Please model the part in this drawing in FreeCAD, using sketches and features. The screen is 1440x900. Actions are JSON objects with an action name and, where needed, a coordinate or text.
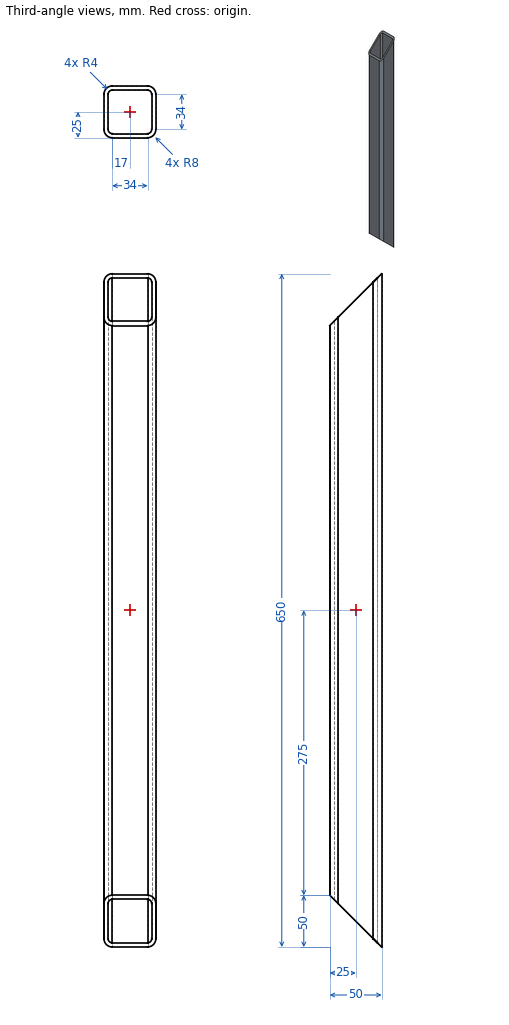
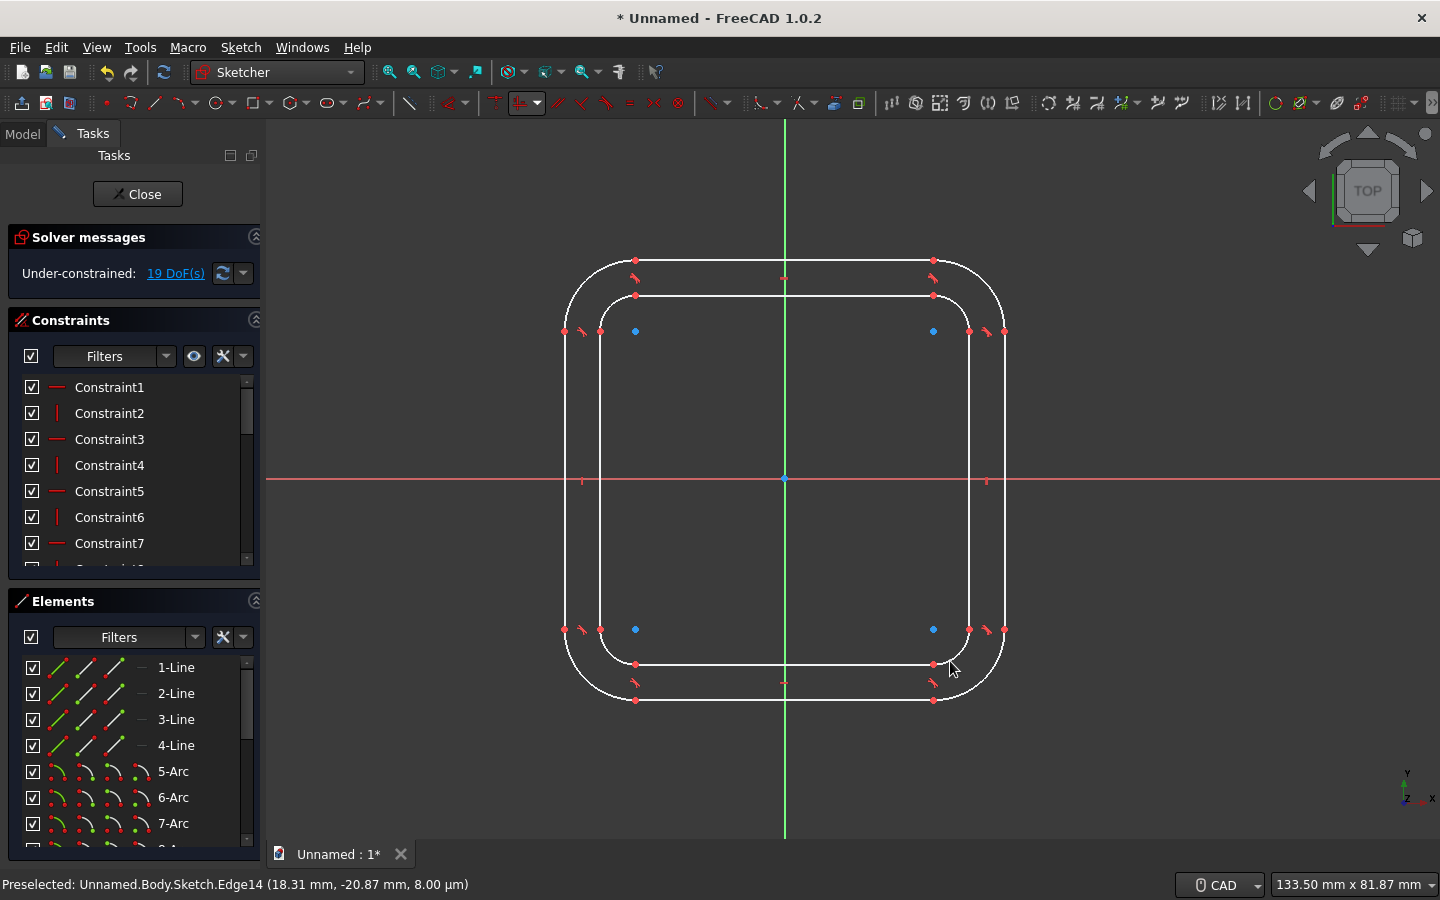
{"action": "left_click", "coordinate": [844, 665]}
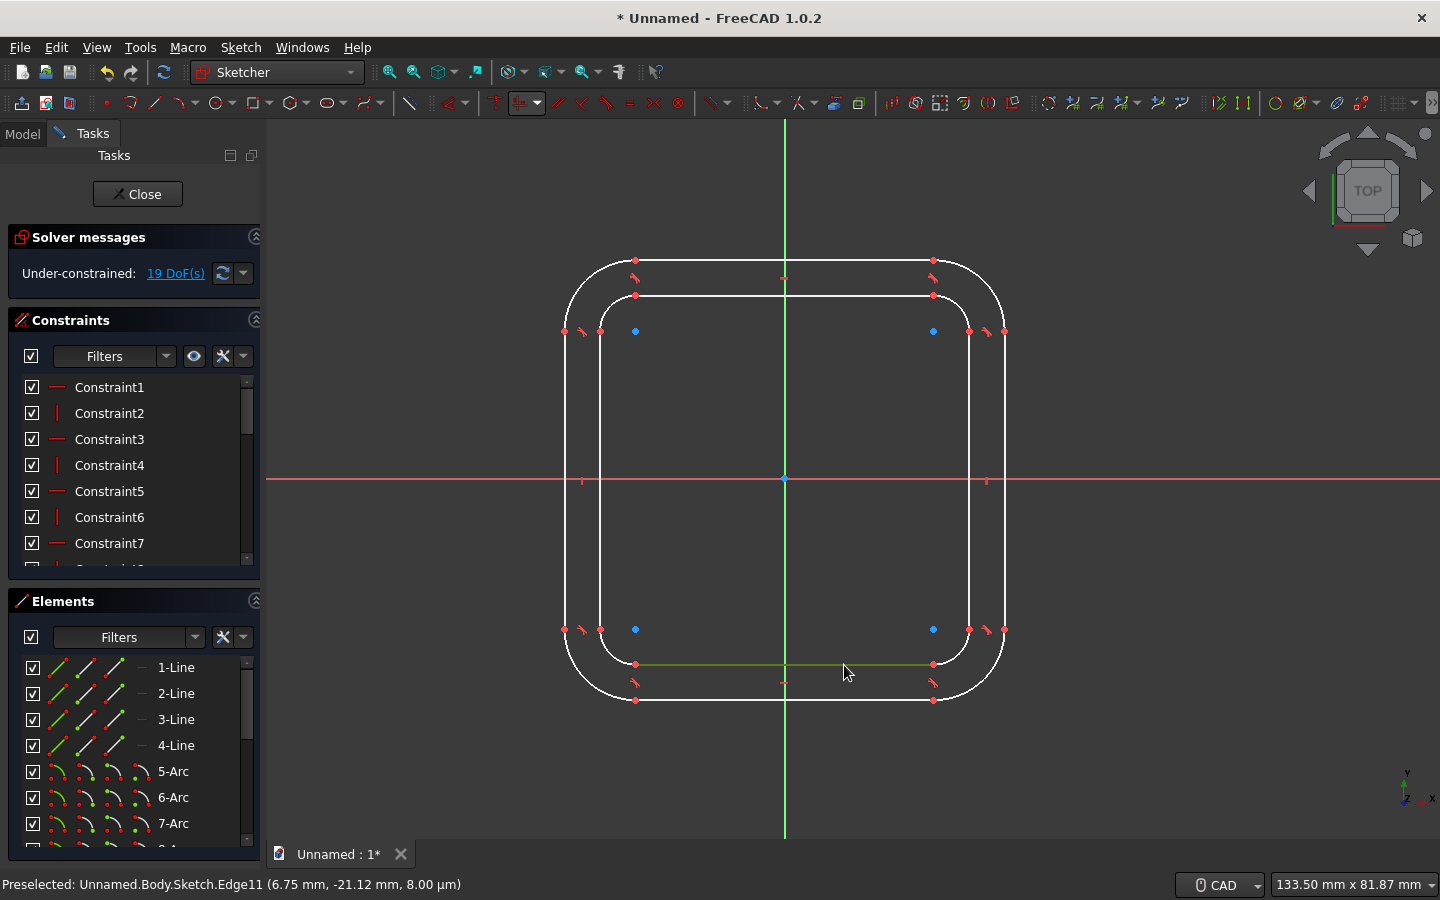
{"action": "left_click", "coordinate": [604, 645]}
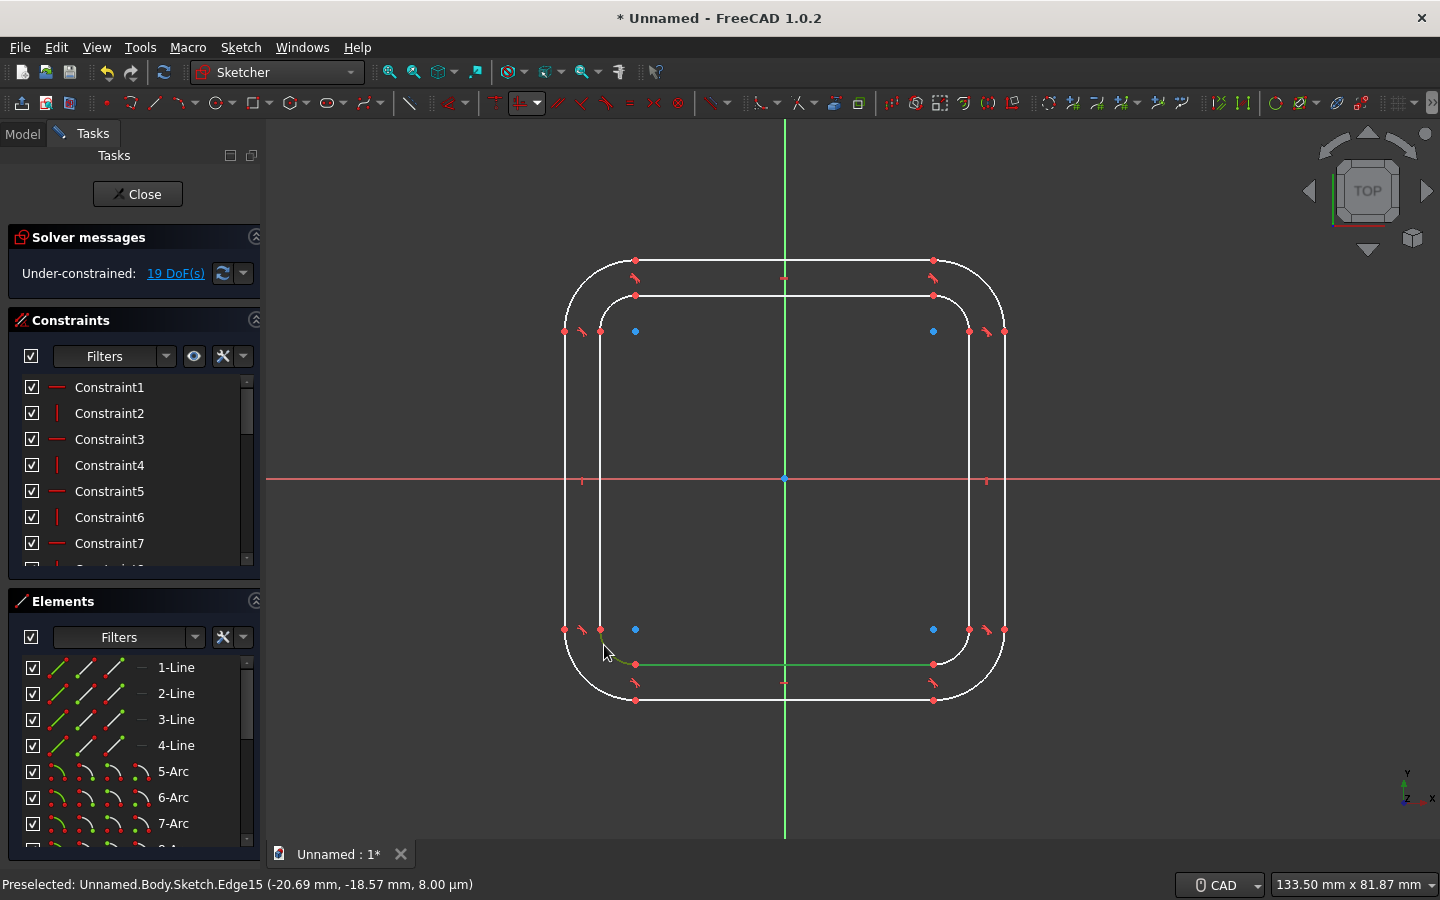
{"action": "left_click", "coordinate": [606, 104]}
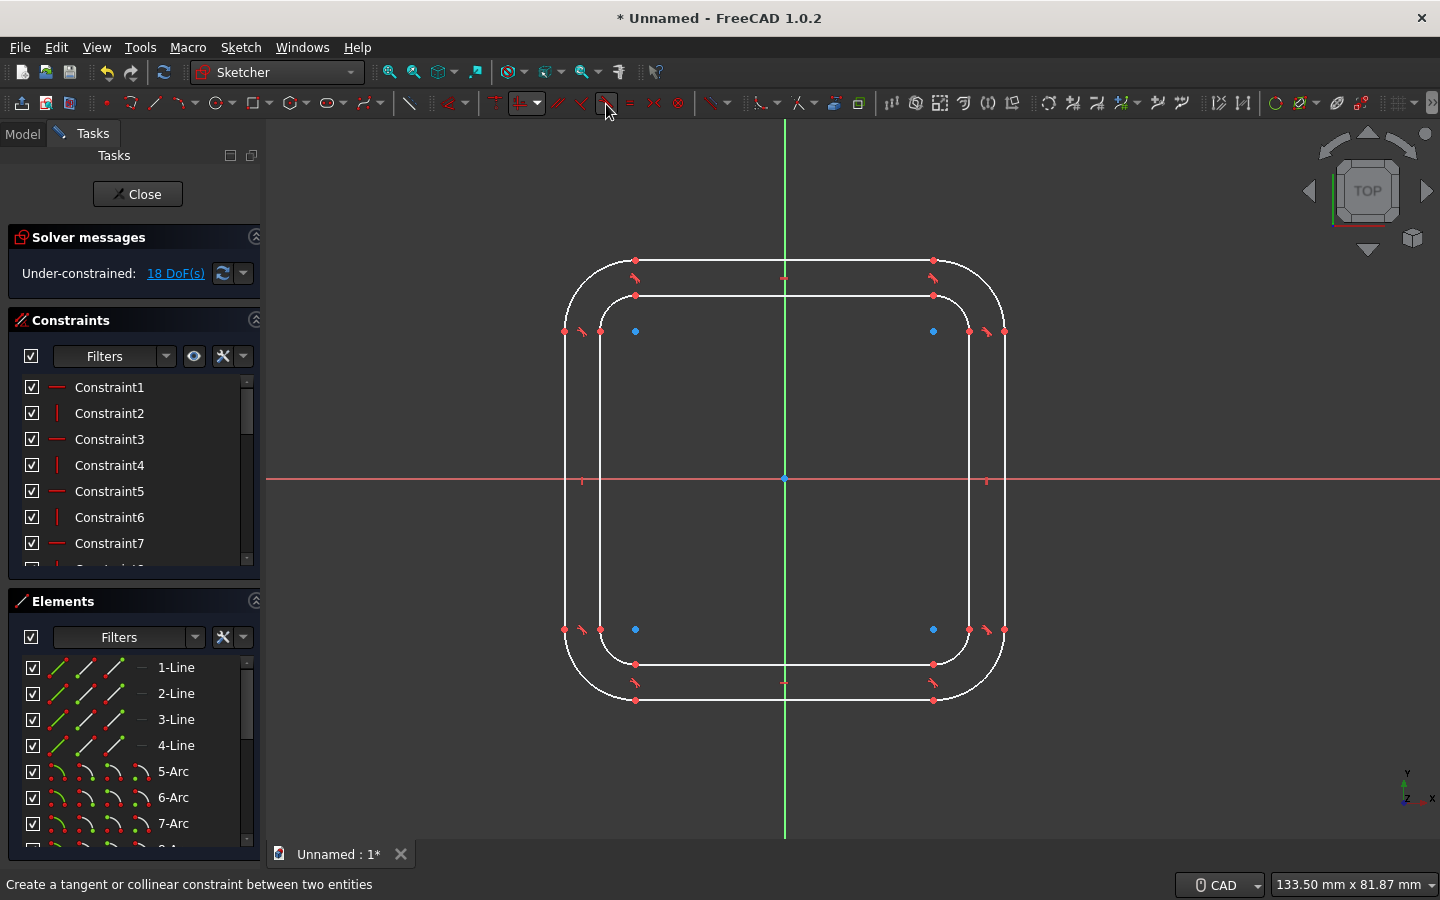
{"action": "left_click", "coordinate": [600, 540]}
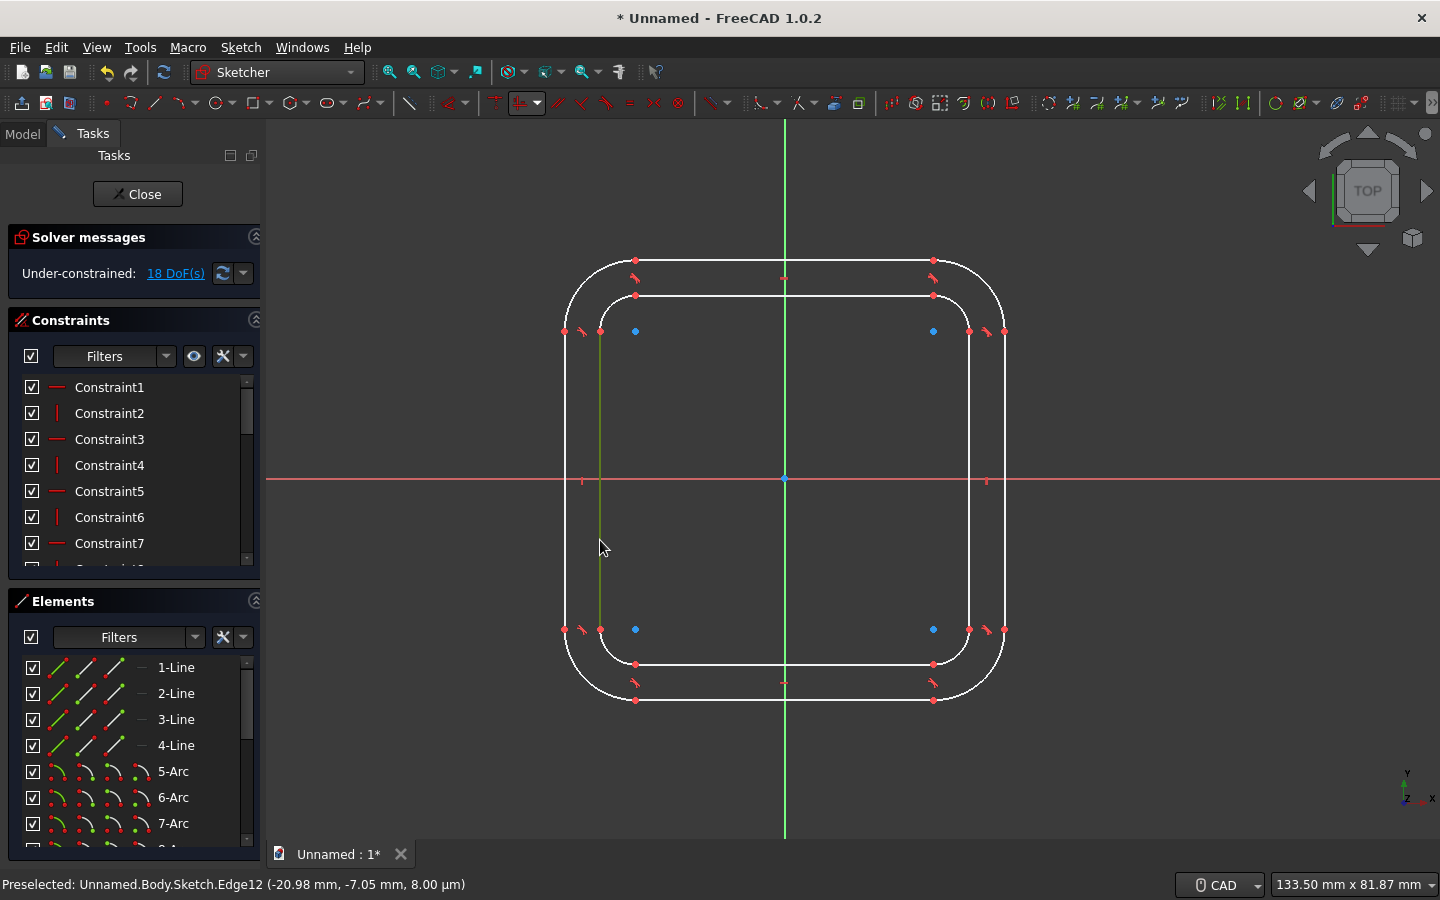
{"action": "left_click", "coordinate": [604, 645]}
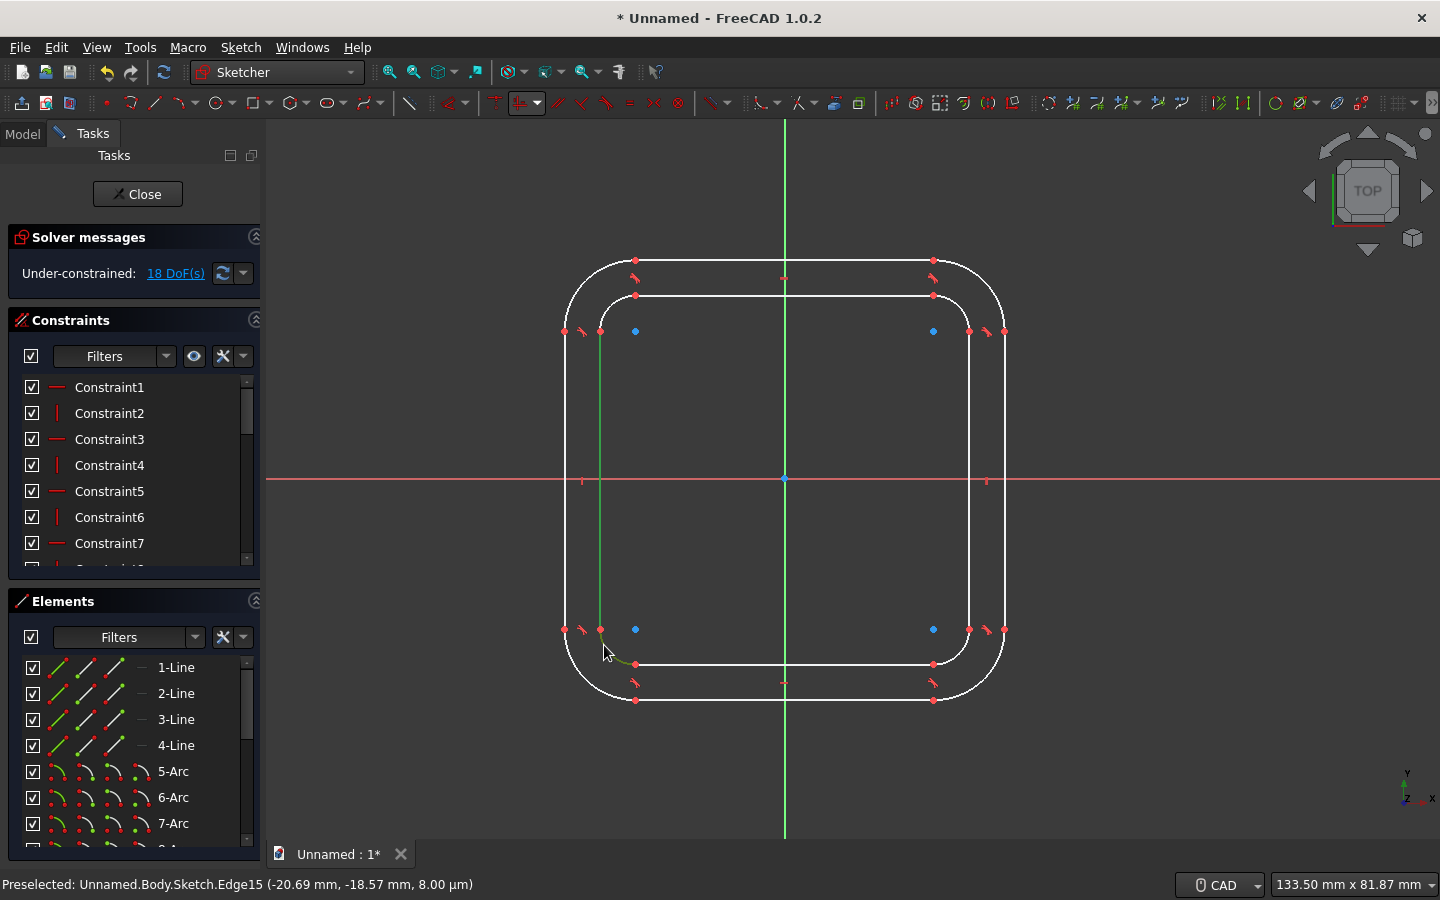
{"action": "key", "text": "t"}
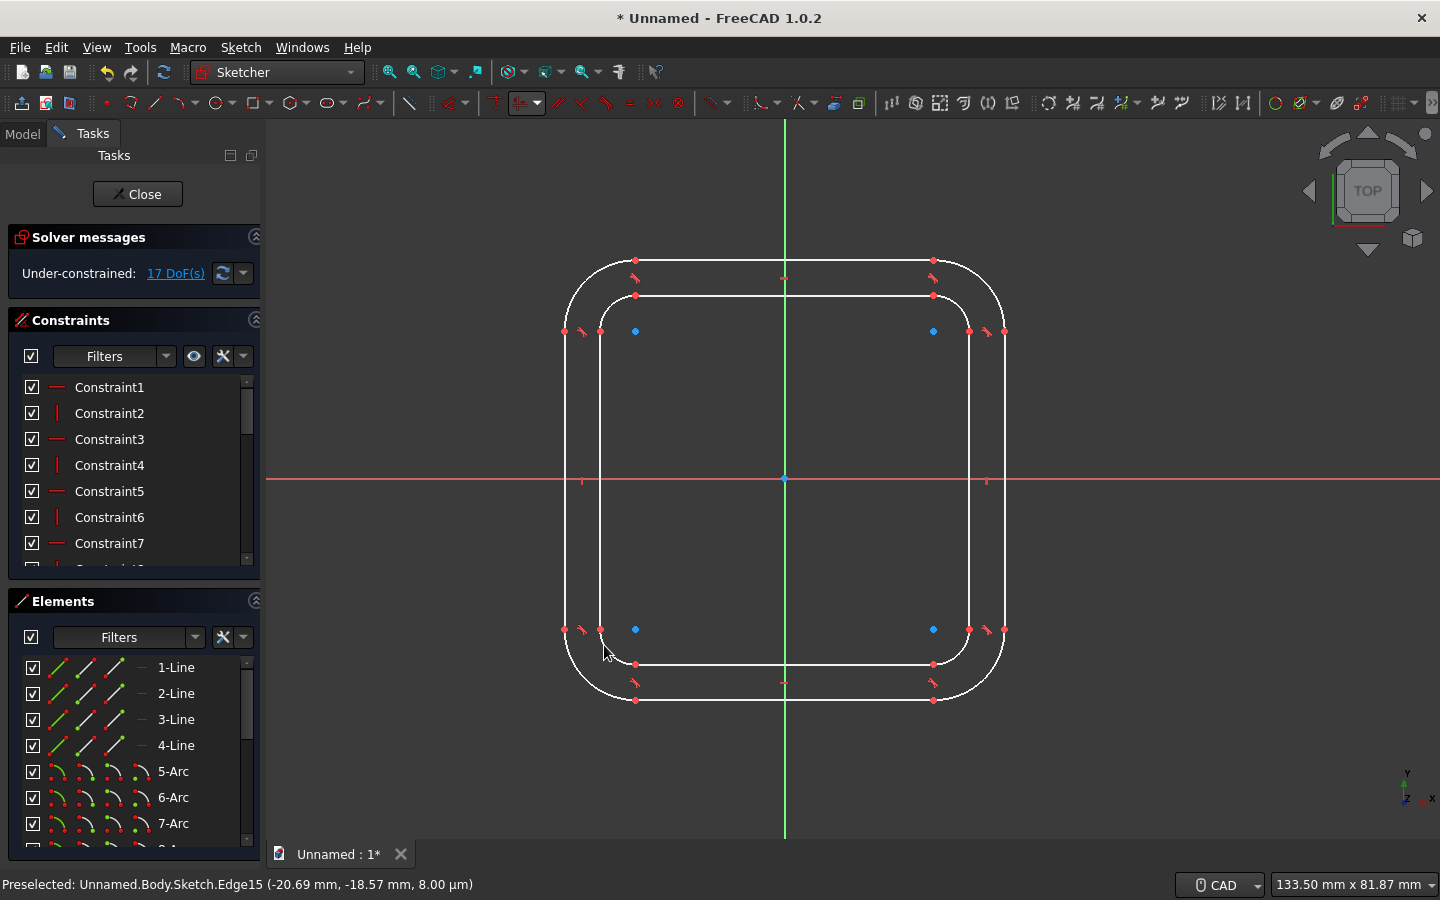
{"action": "left_click", "coordinate": [600, 540]}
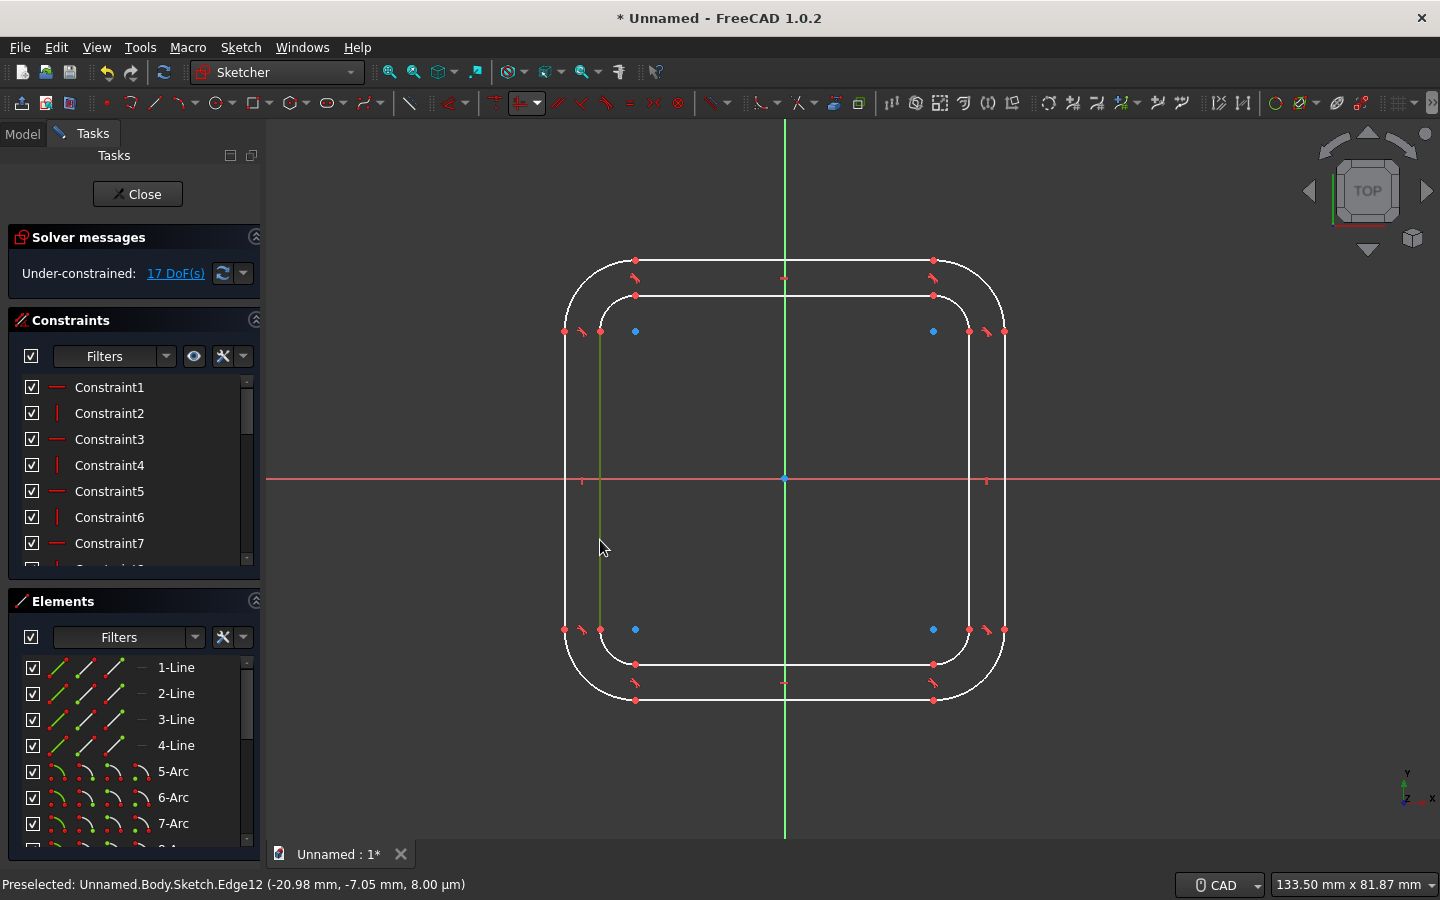
{"action": "left_click", "coordinate": [619, 300]}